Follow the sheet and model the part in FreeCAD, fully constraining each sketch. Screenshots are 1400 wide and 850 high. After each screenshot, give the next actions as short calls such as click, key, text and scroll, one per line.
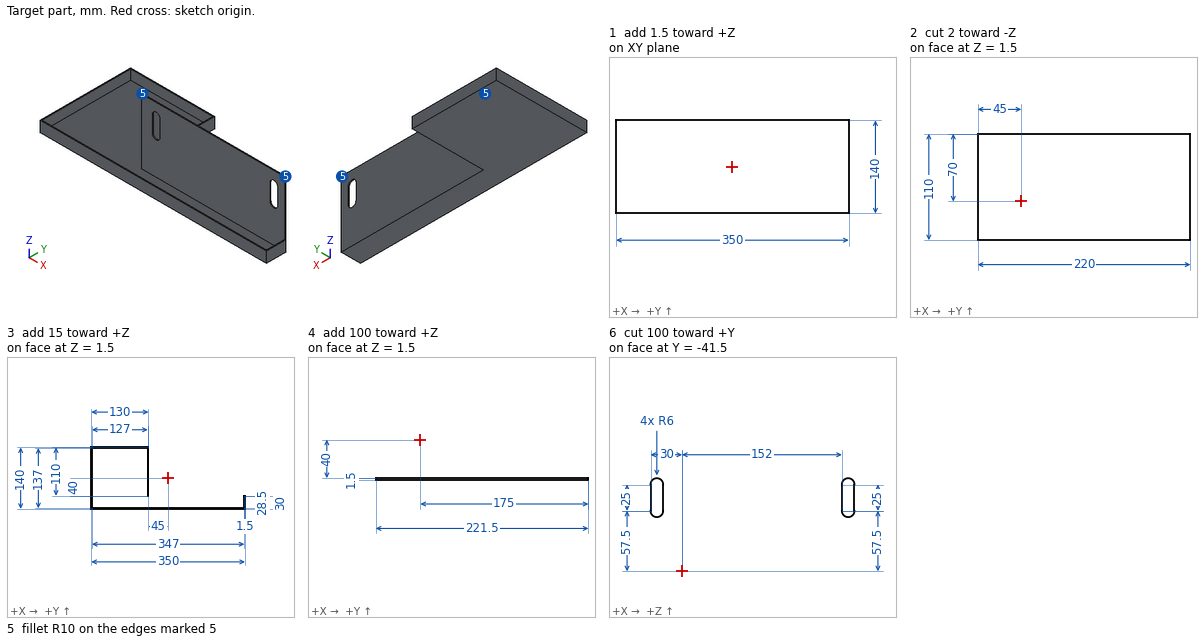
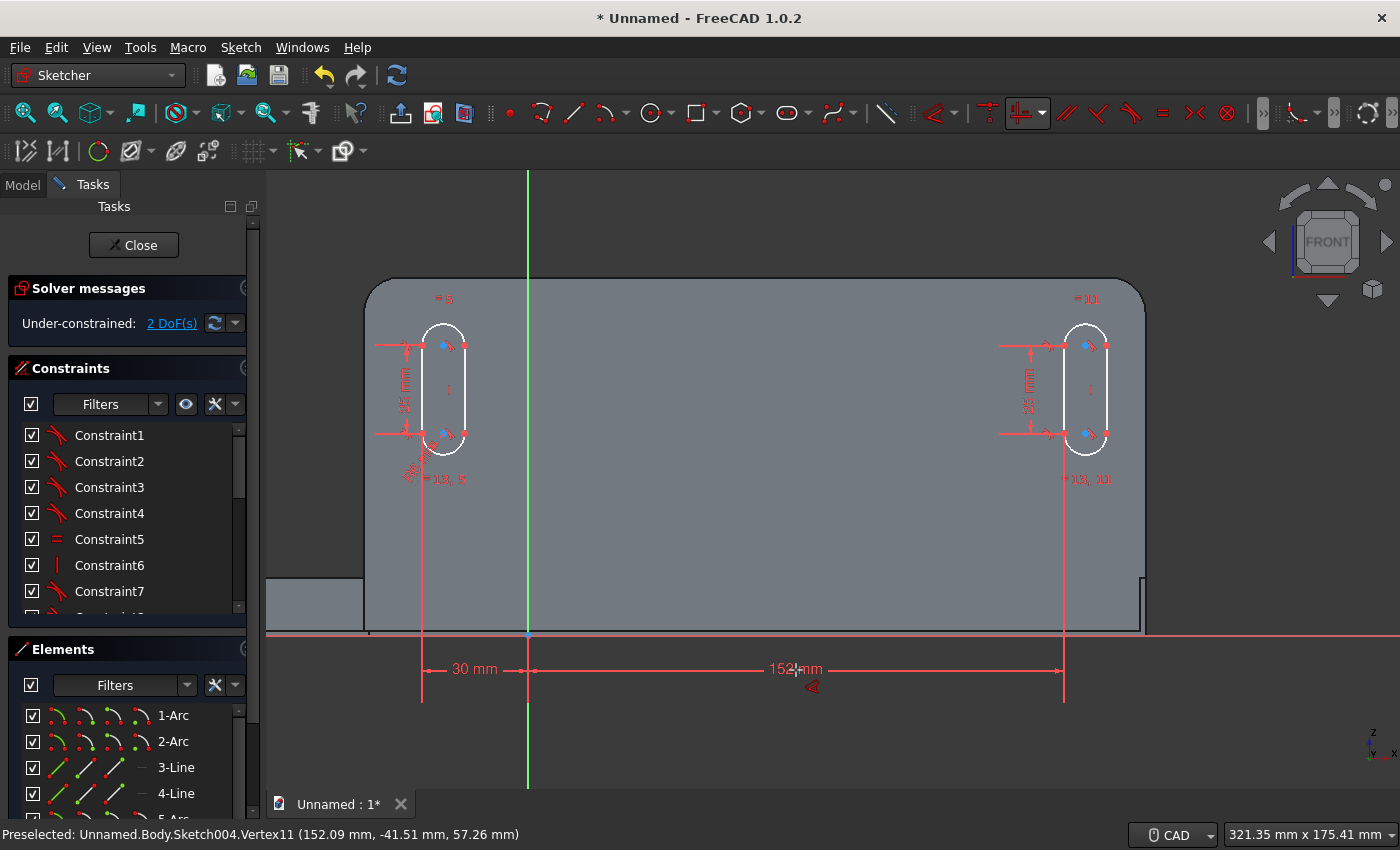
click(422, 434)
click(388, 535)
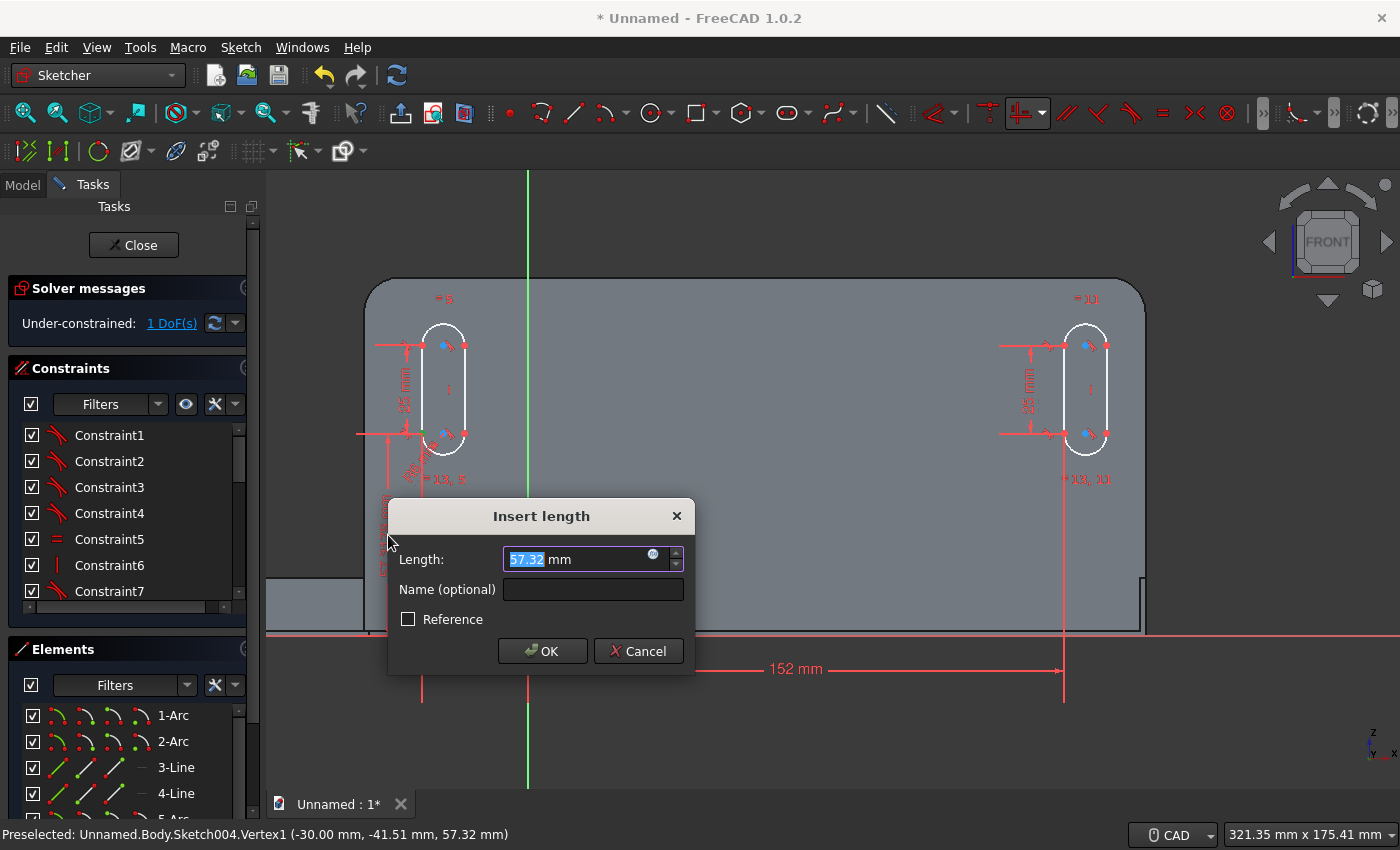
text(57.5)
key(Return)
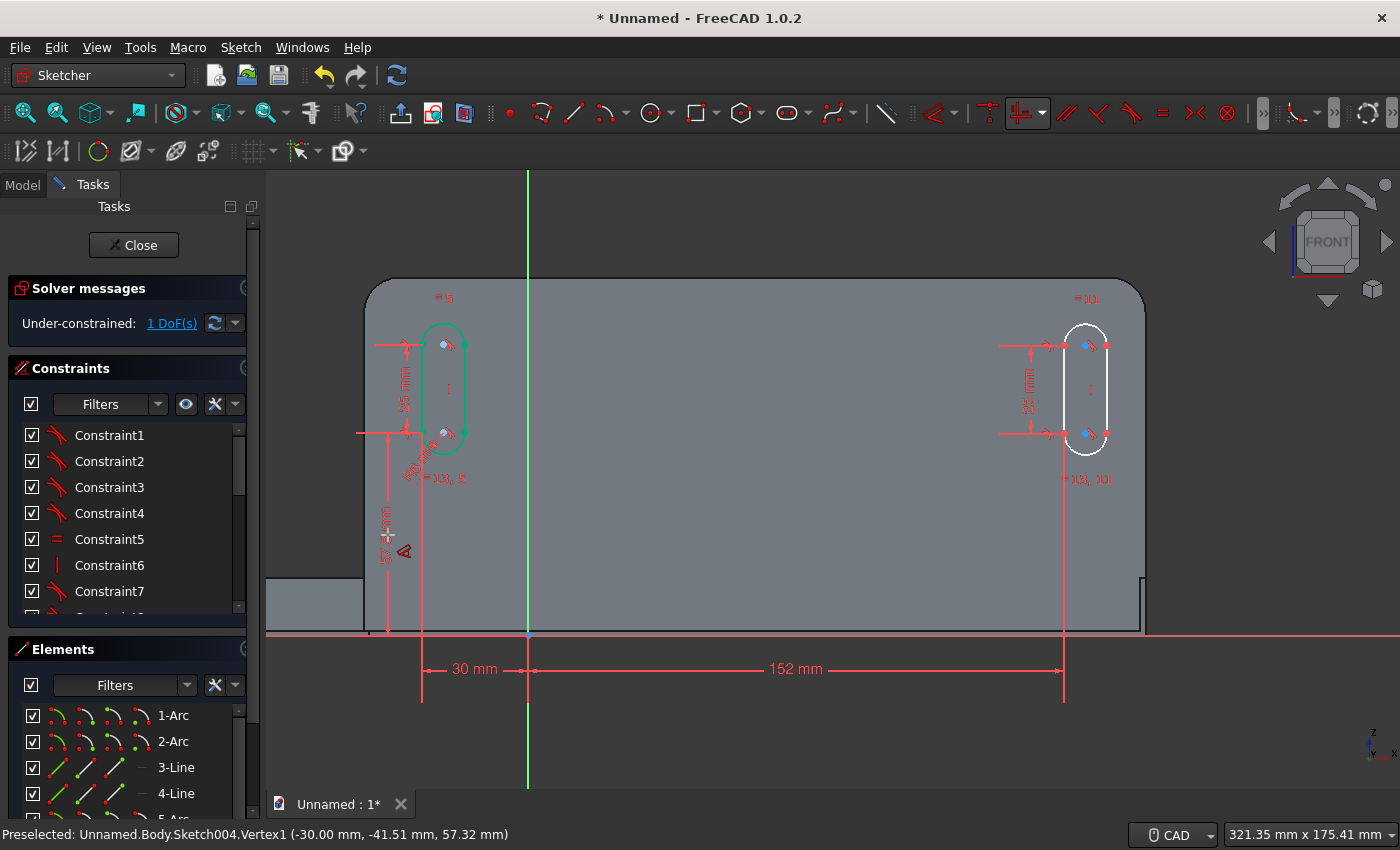
click(1064, 434)
click(1098, 535)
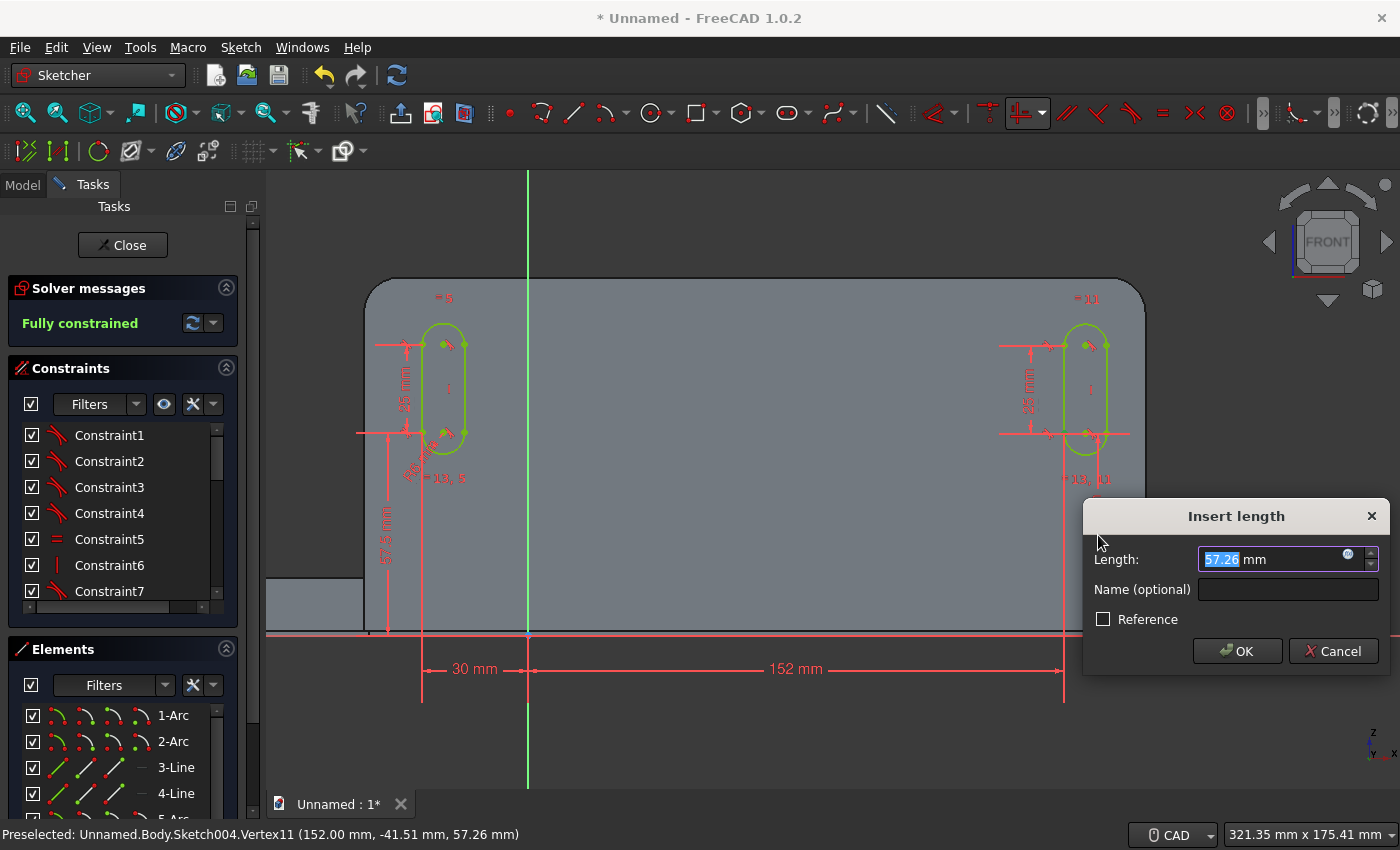
text(57.5)
key(Return)
key(Escape)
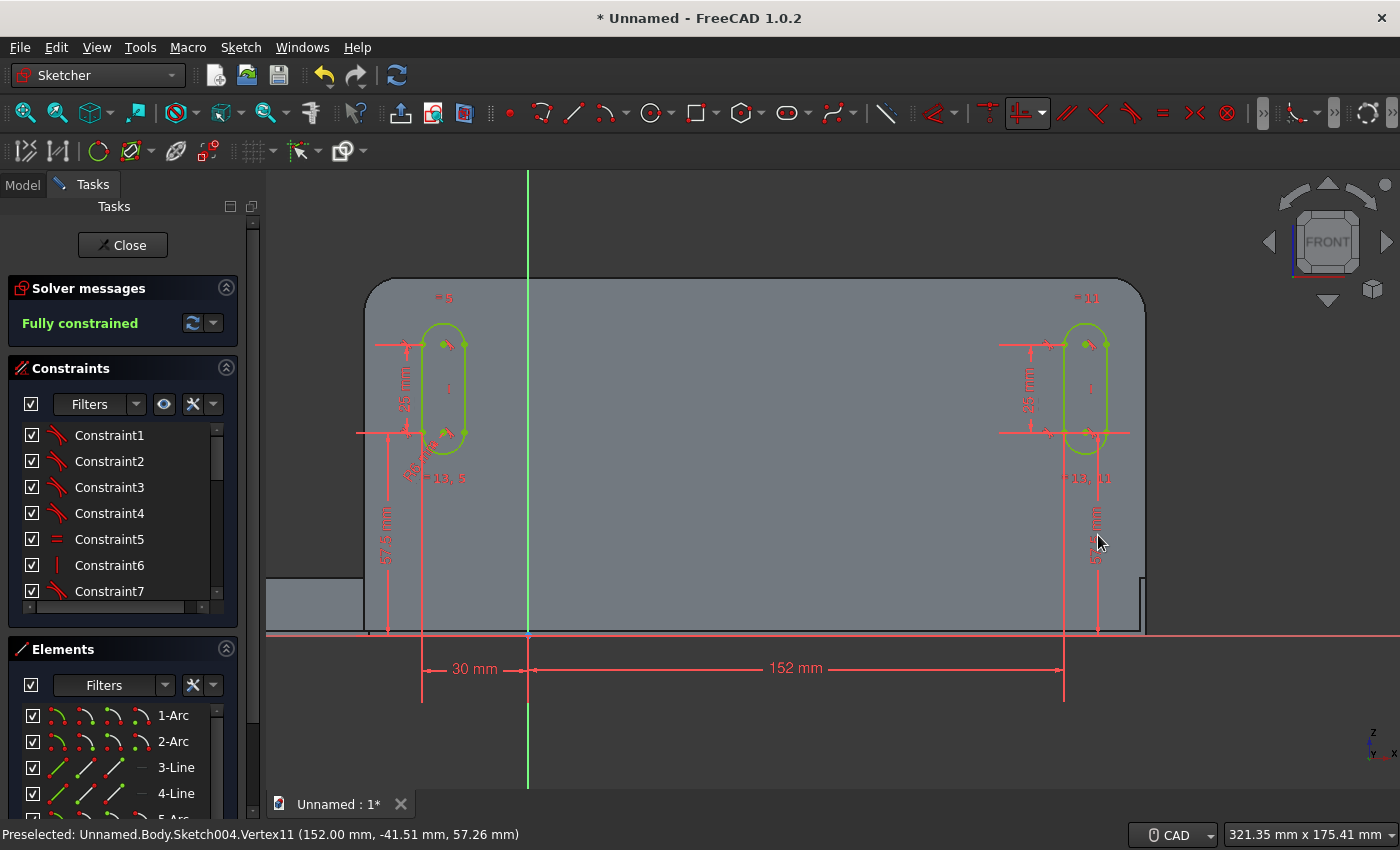
click(123, 245)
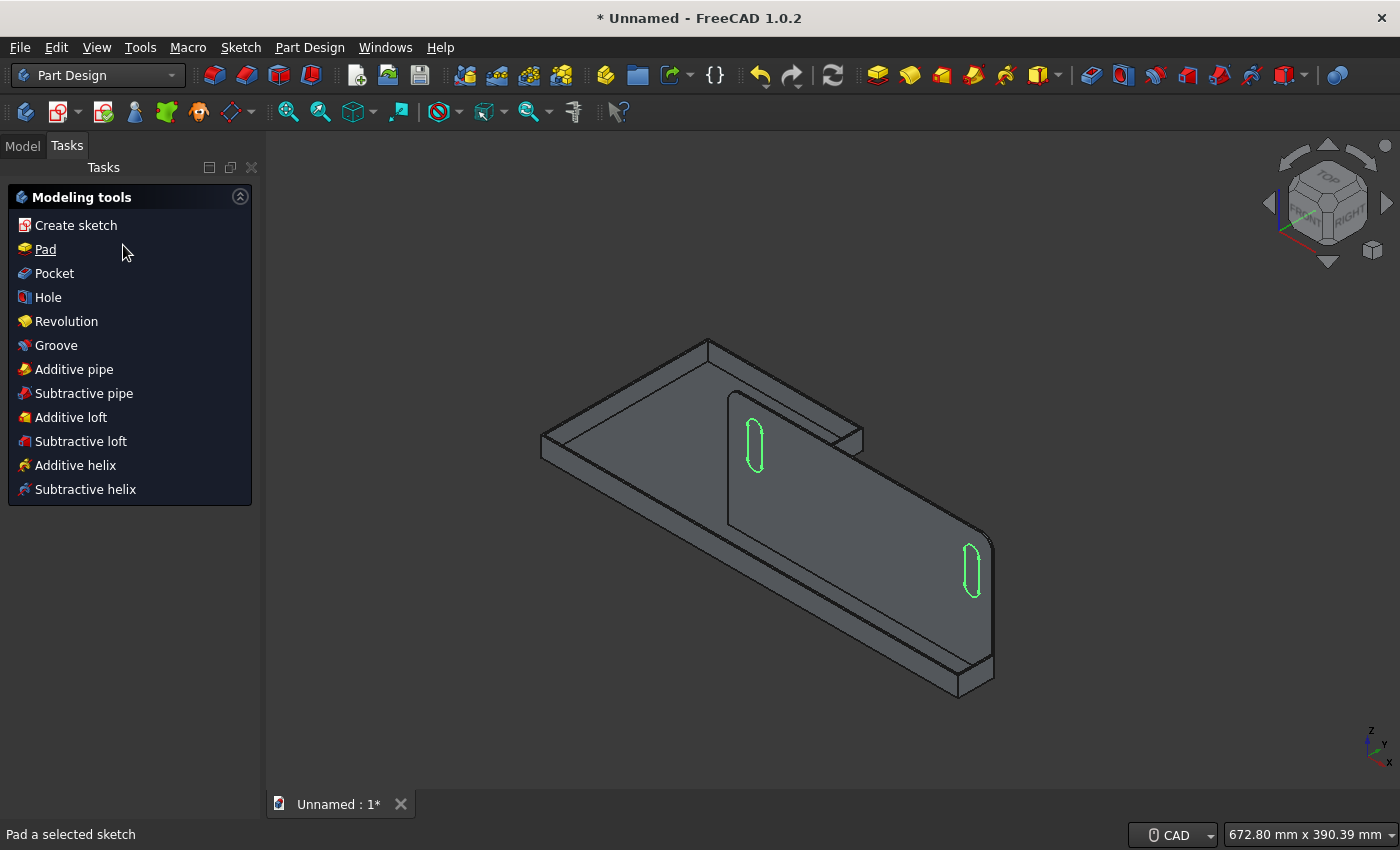
click(1092, 76)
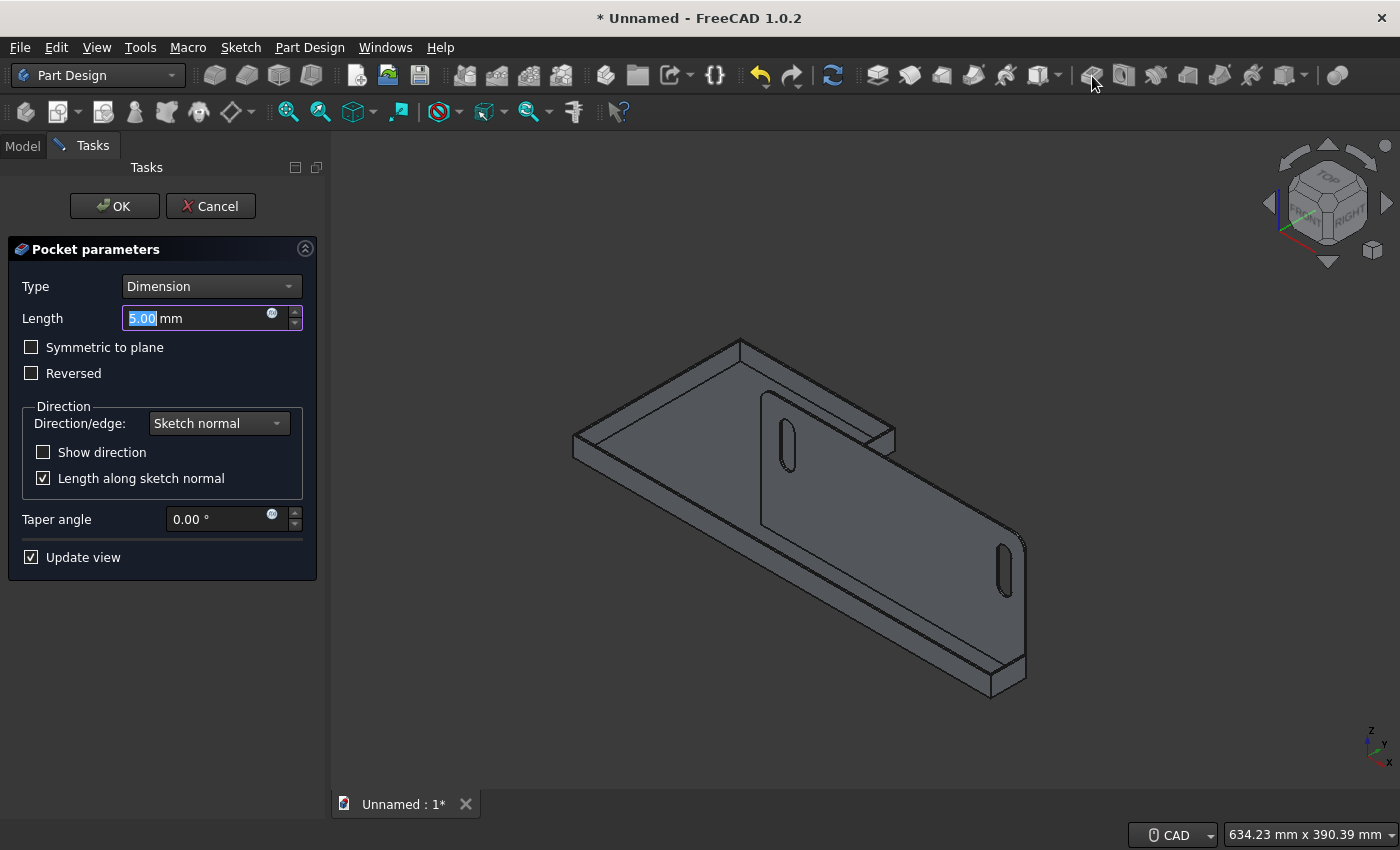
text(100)
key(Tab)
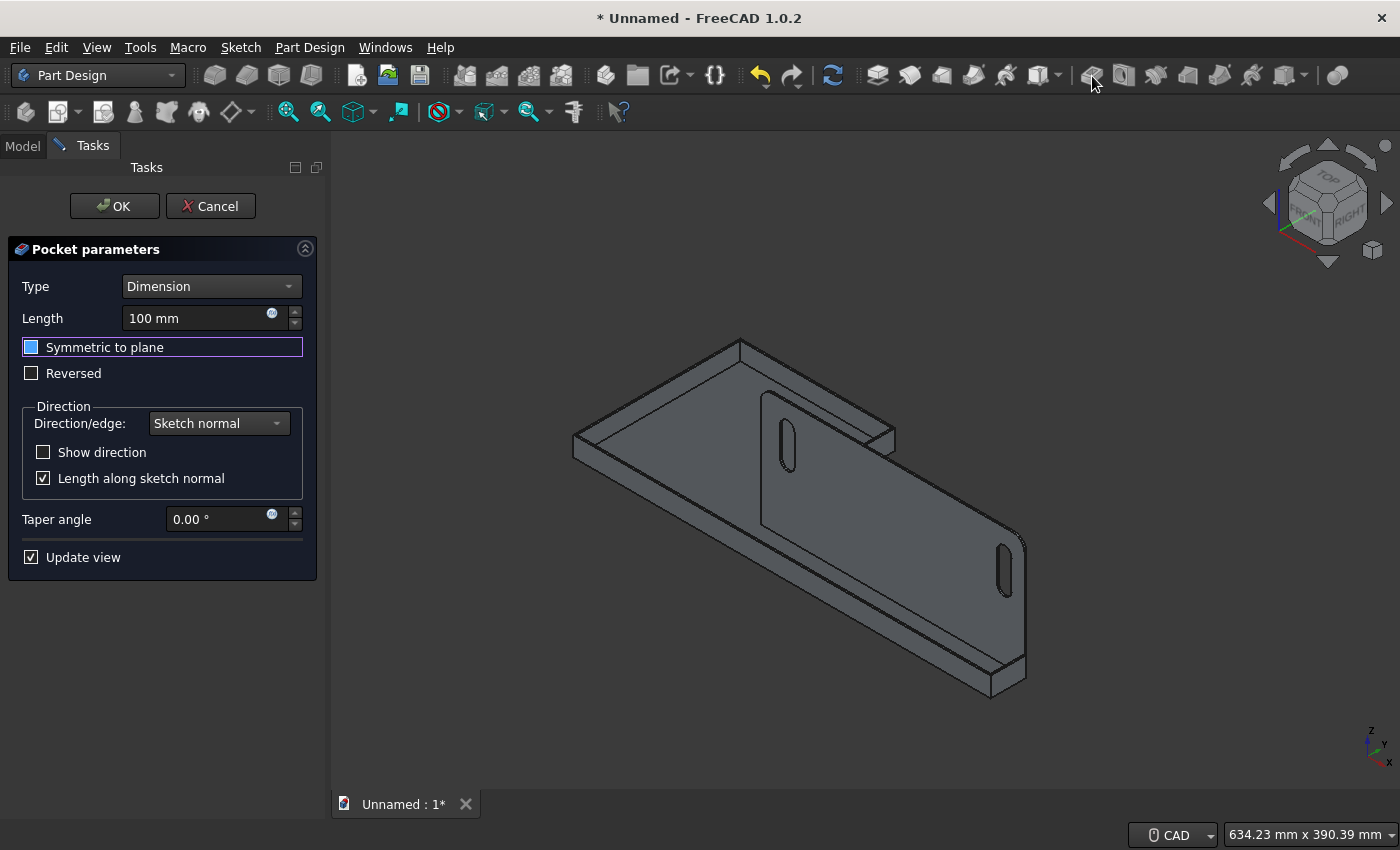
click(115, 206)